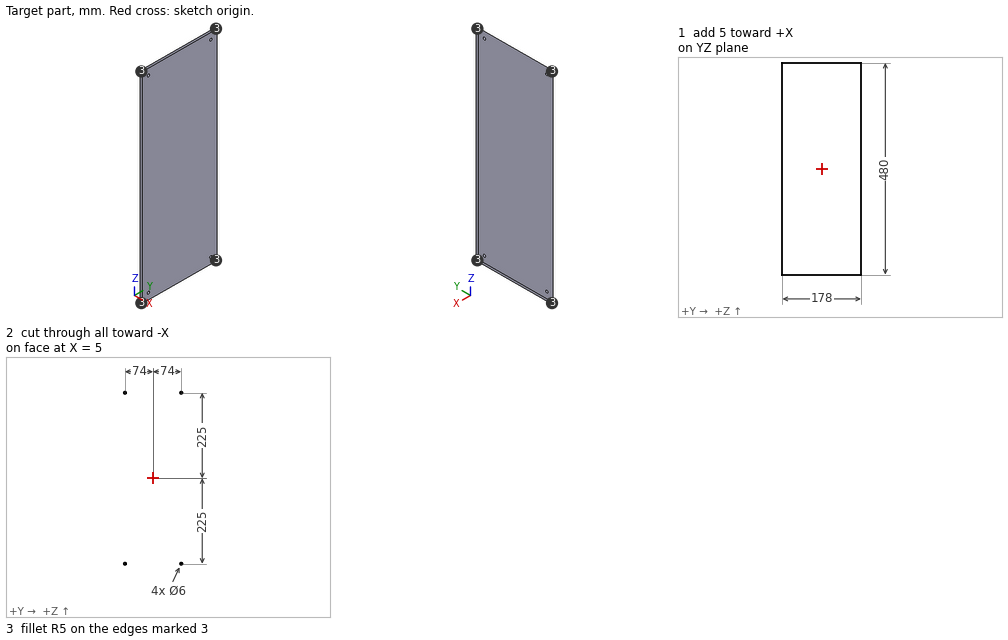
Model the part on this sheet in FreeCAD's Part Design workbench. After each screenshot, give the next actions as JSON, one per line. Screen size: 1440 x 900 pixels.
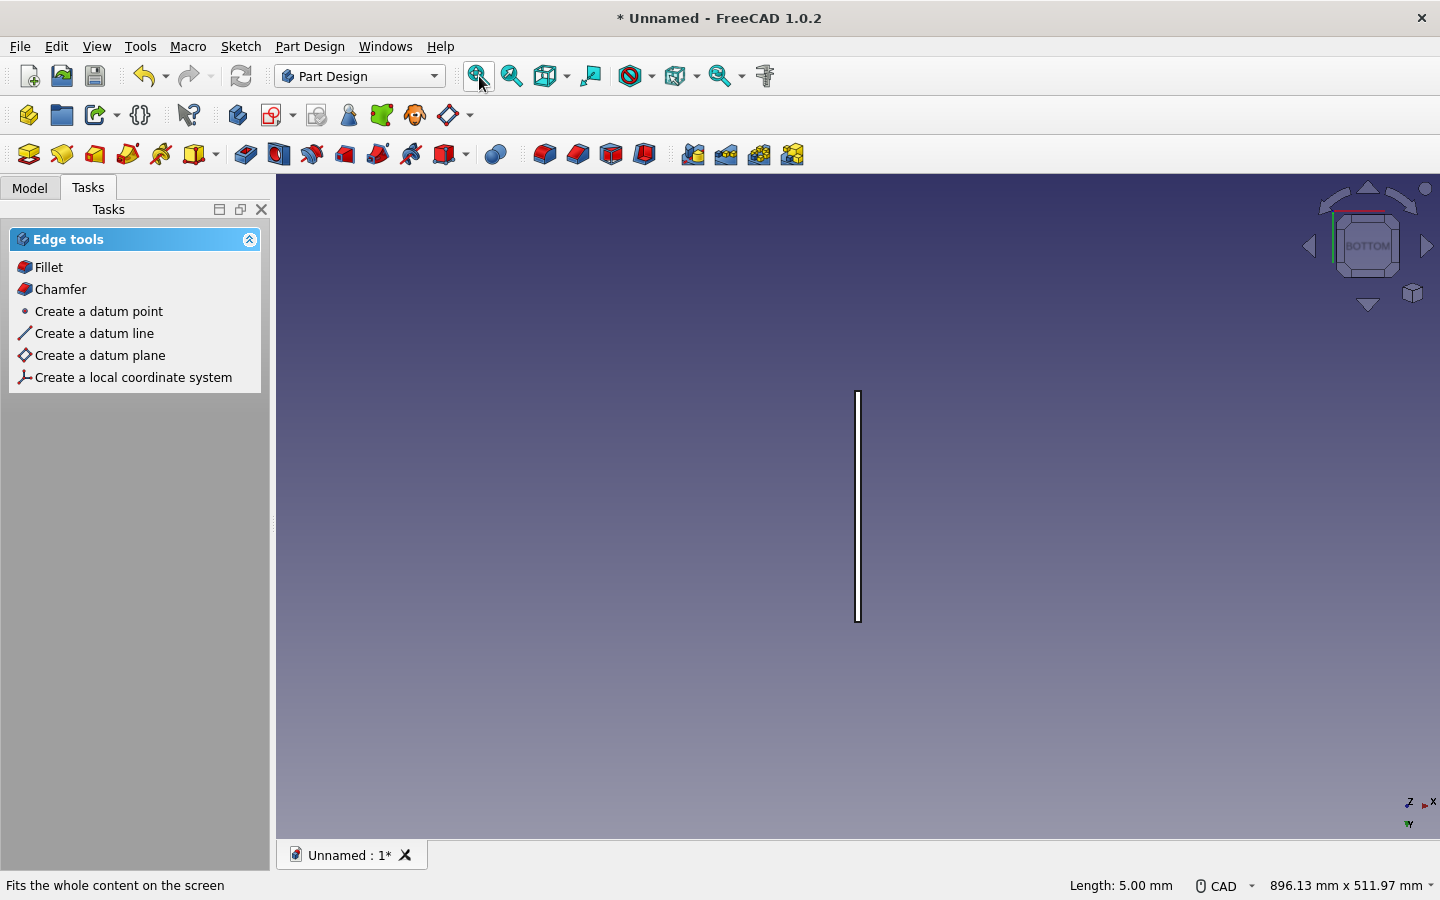
{"action": "scroll", "coordinate": [858, 621], "scroll_direction": "up", "scroll_amount": 10}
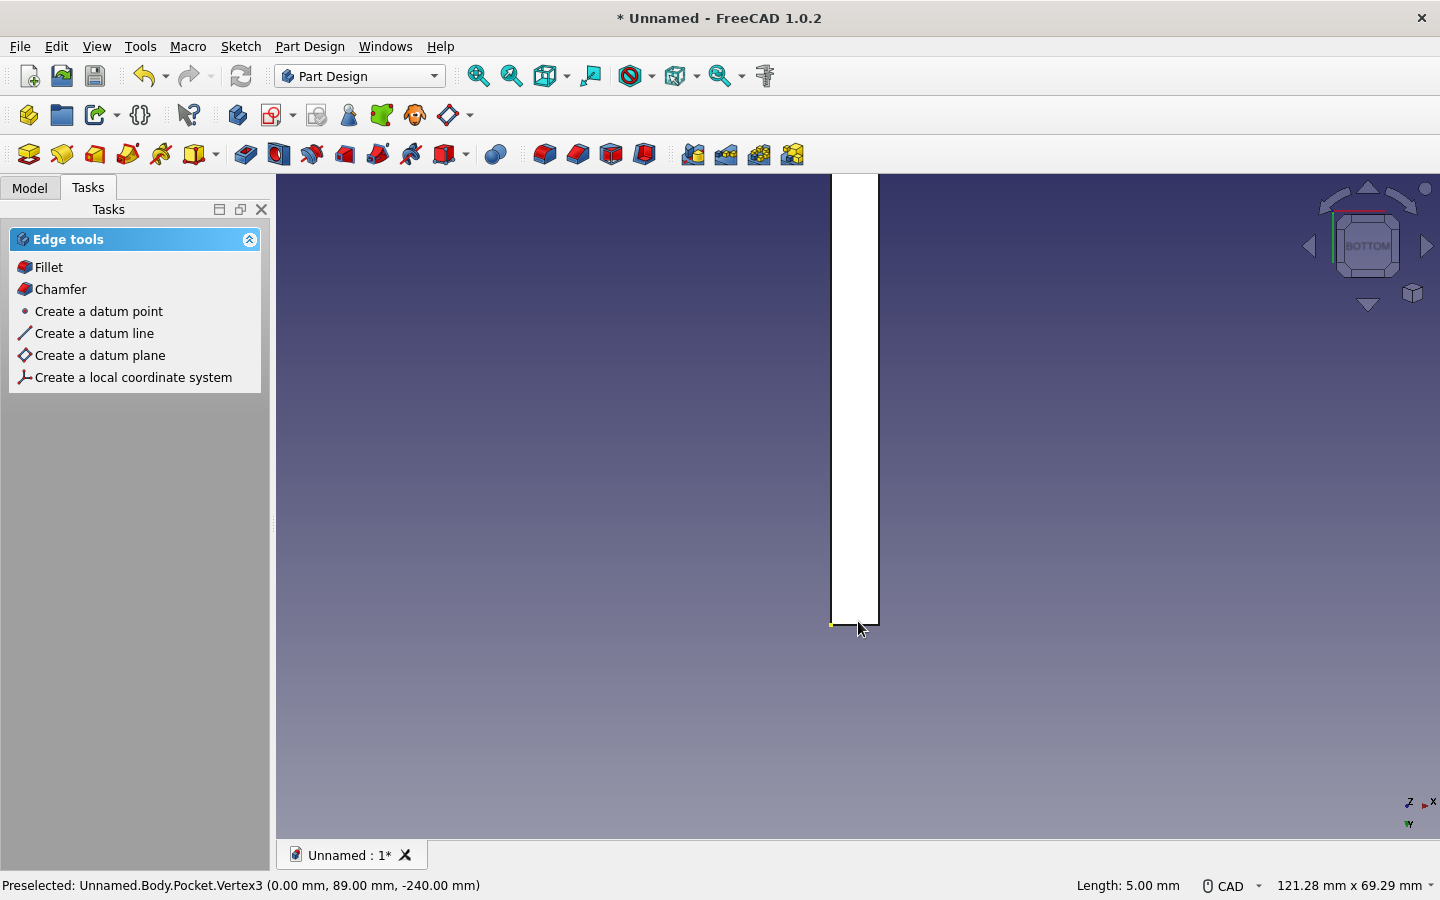
{"action": "left_click", "coordinate": [855, 624], "text": "ctrl"}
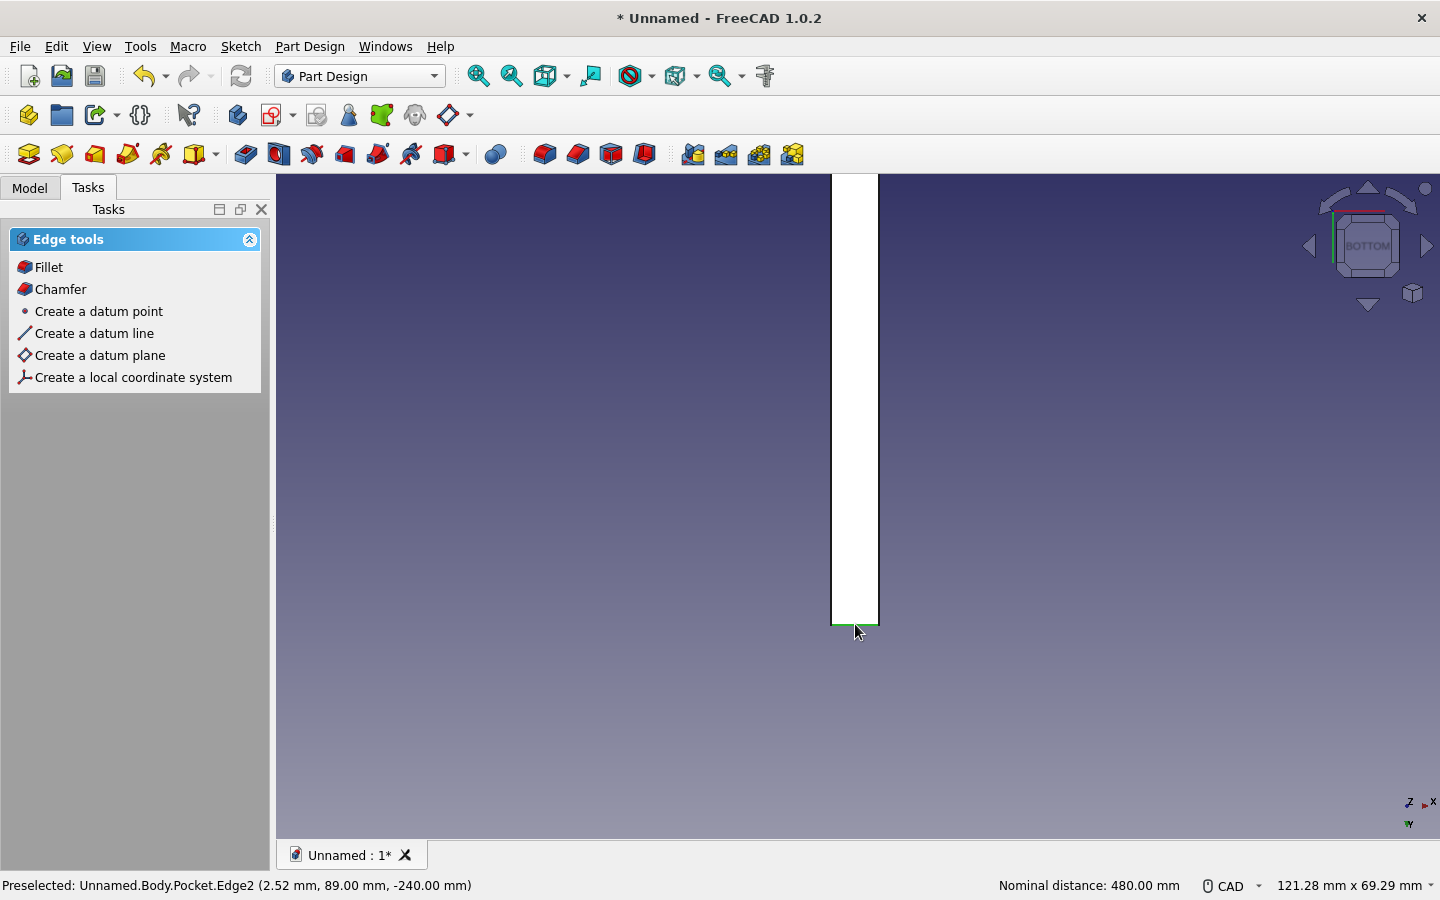
{"action": "left_click", "coordinate": [479, 76]}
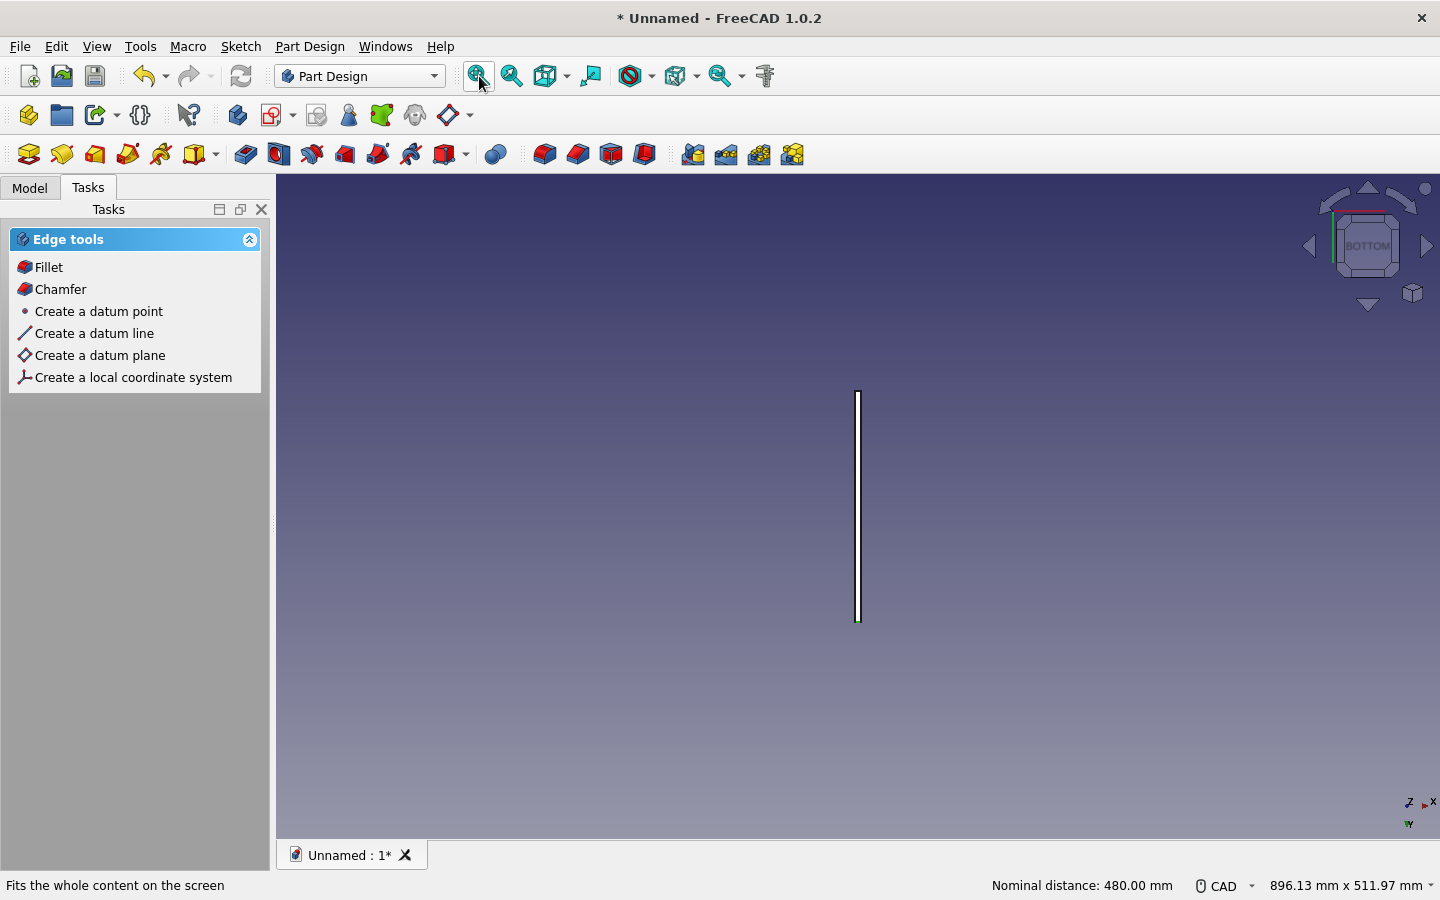
{"action": "key", "text": "4"}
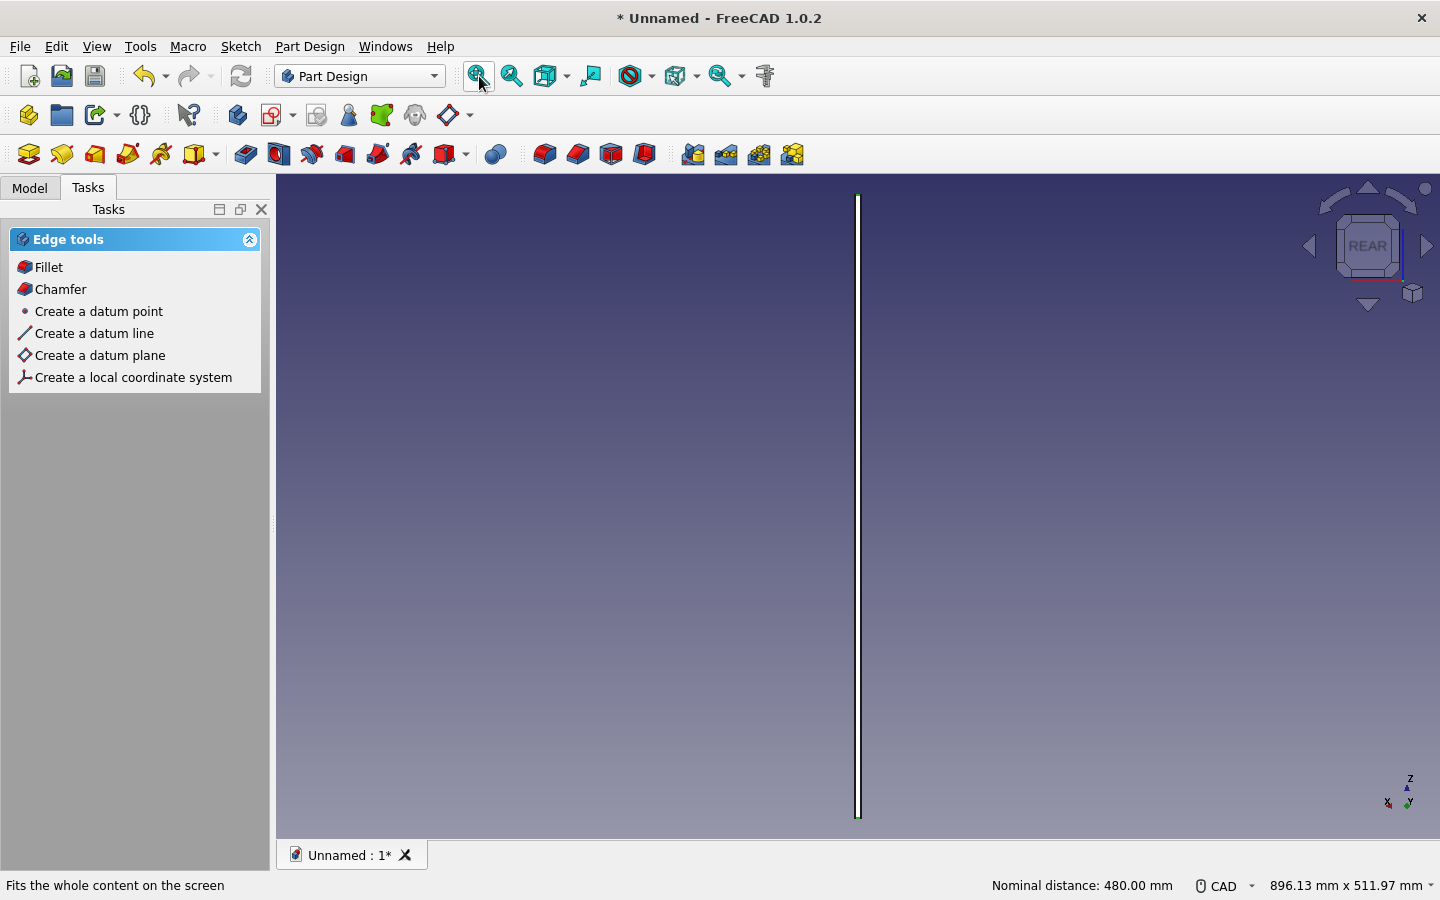
{"action": "key", "text": "6"}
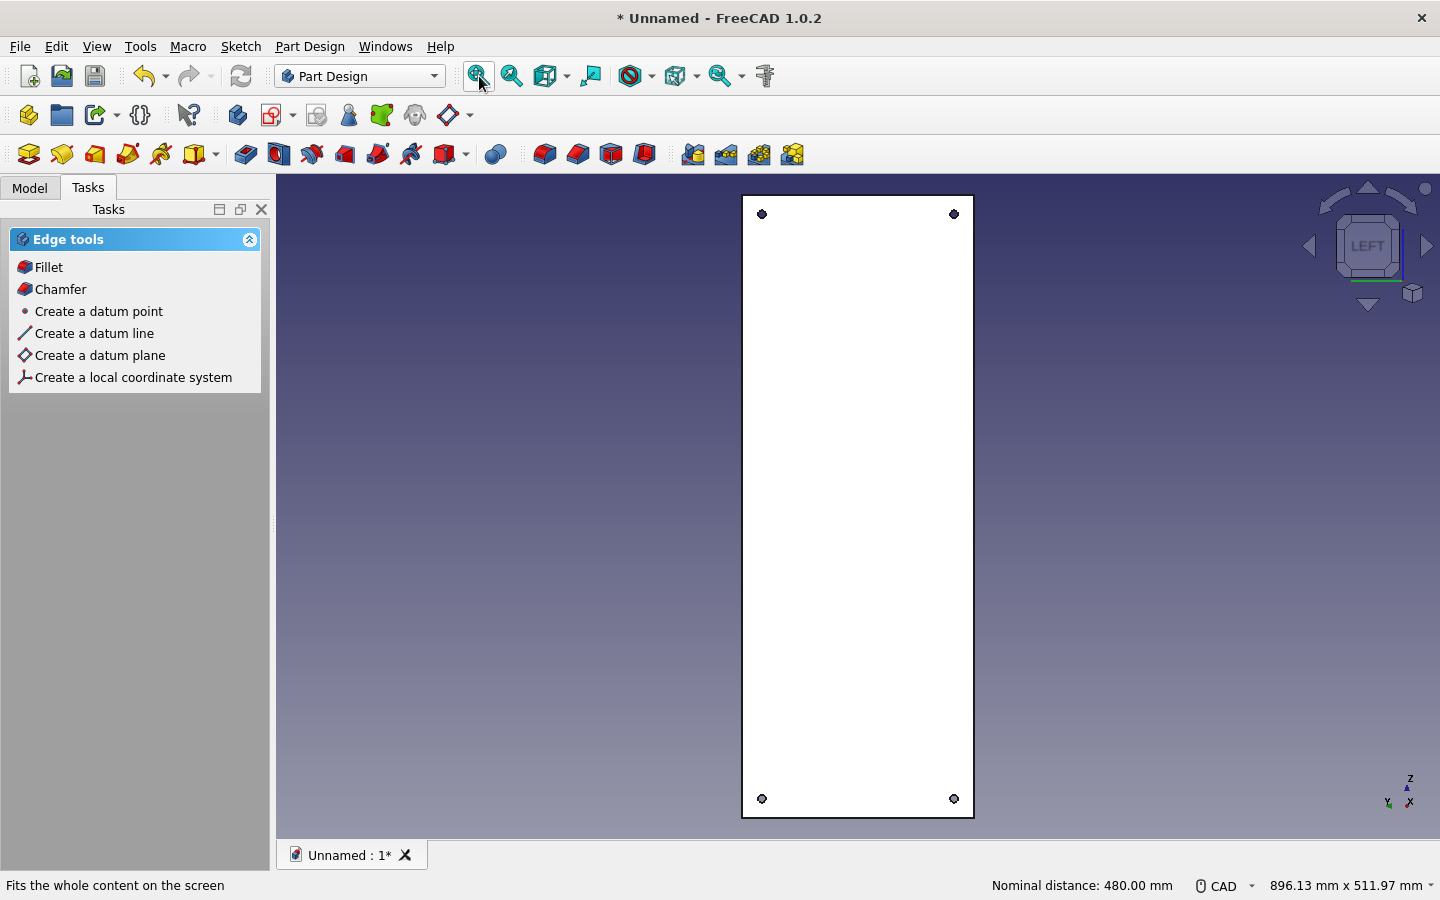
{"action": "key", "text": "v 3"}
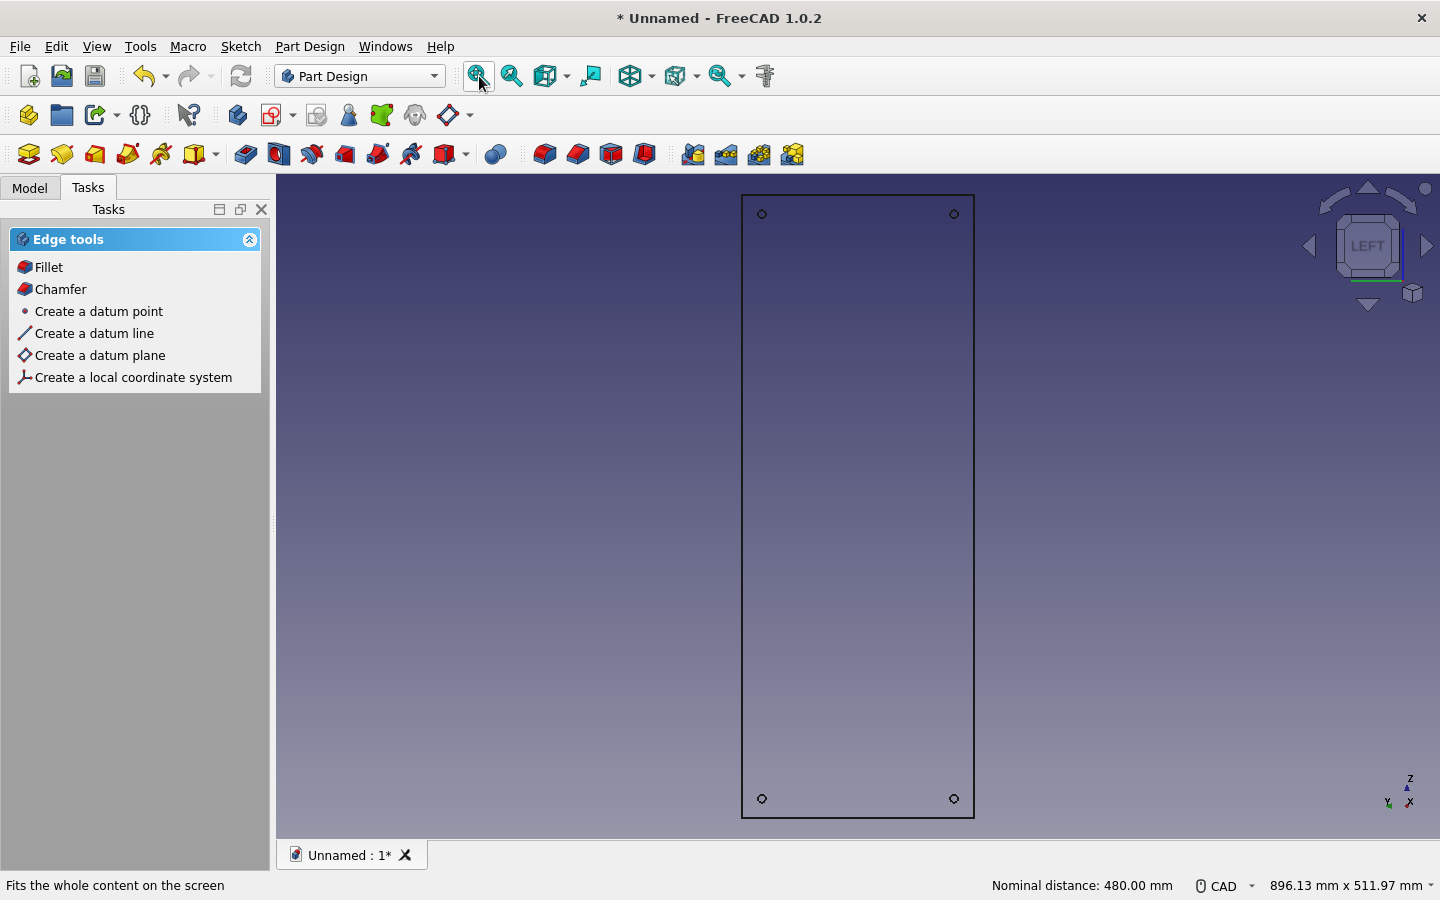
{"action": "key", "text": "0"}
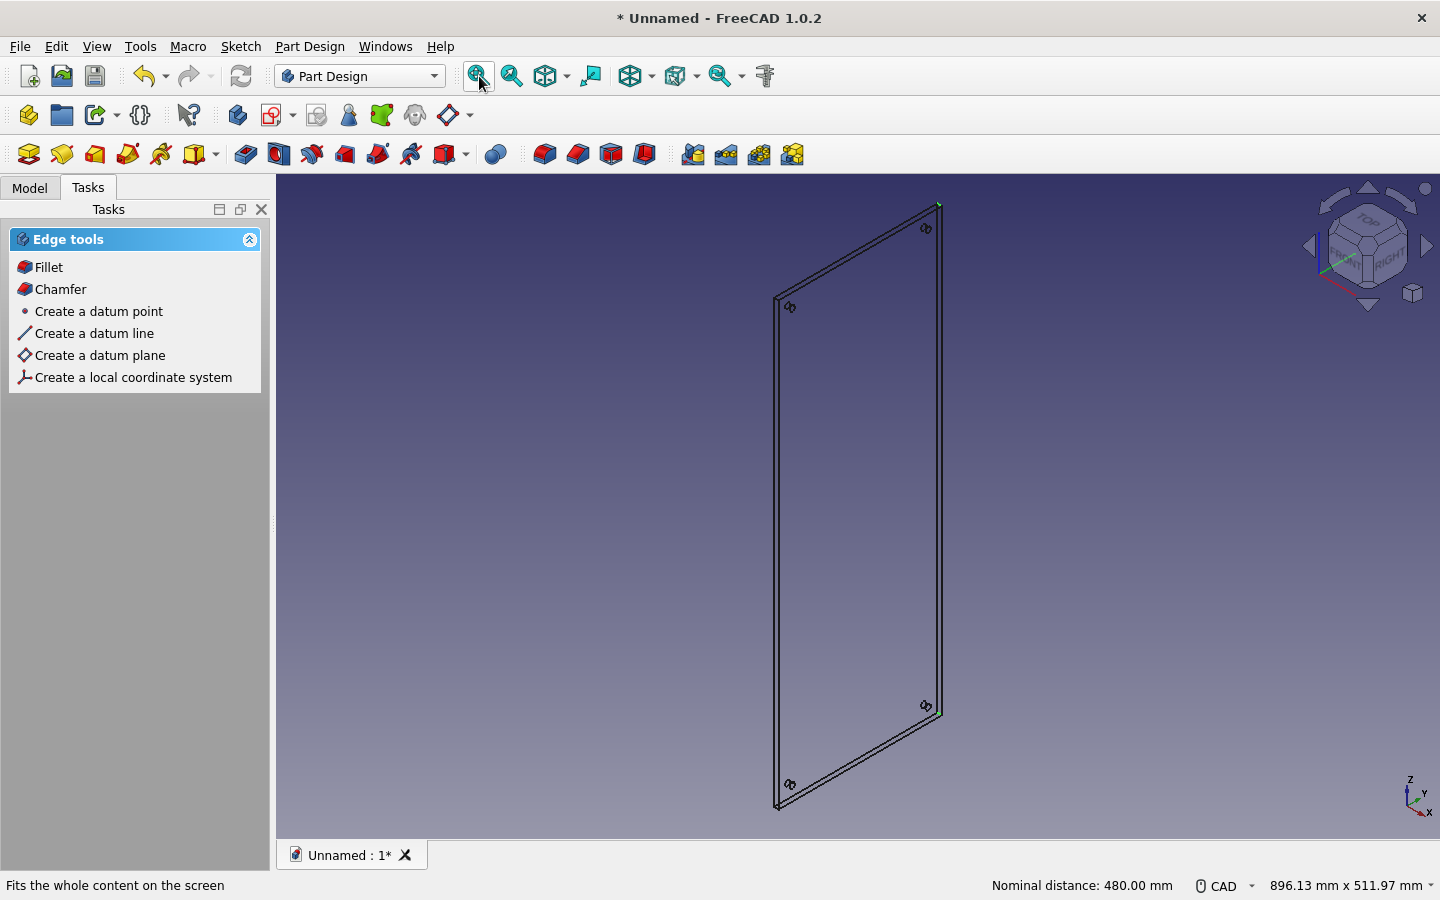
{"action": "scroll", "coordinate": [776, 807], "scroll_direction": "up", "scroll_amount": 10}